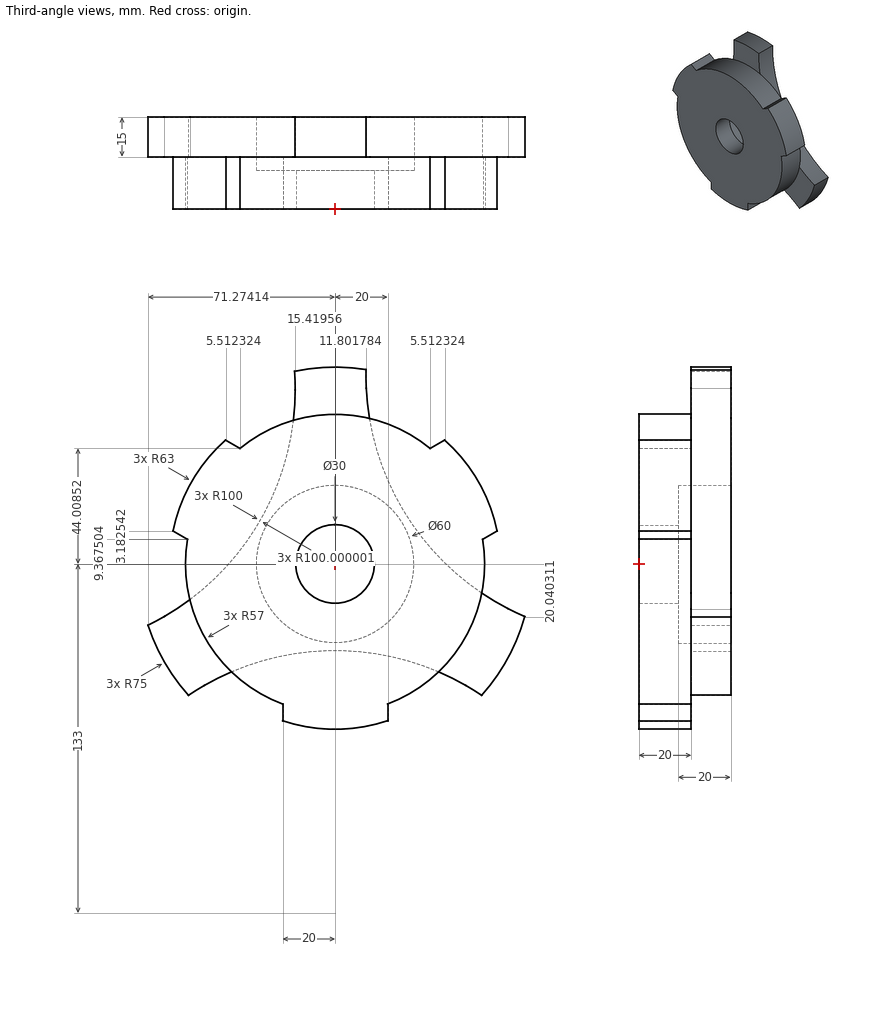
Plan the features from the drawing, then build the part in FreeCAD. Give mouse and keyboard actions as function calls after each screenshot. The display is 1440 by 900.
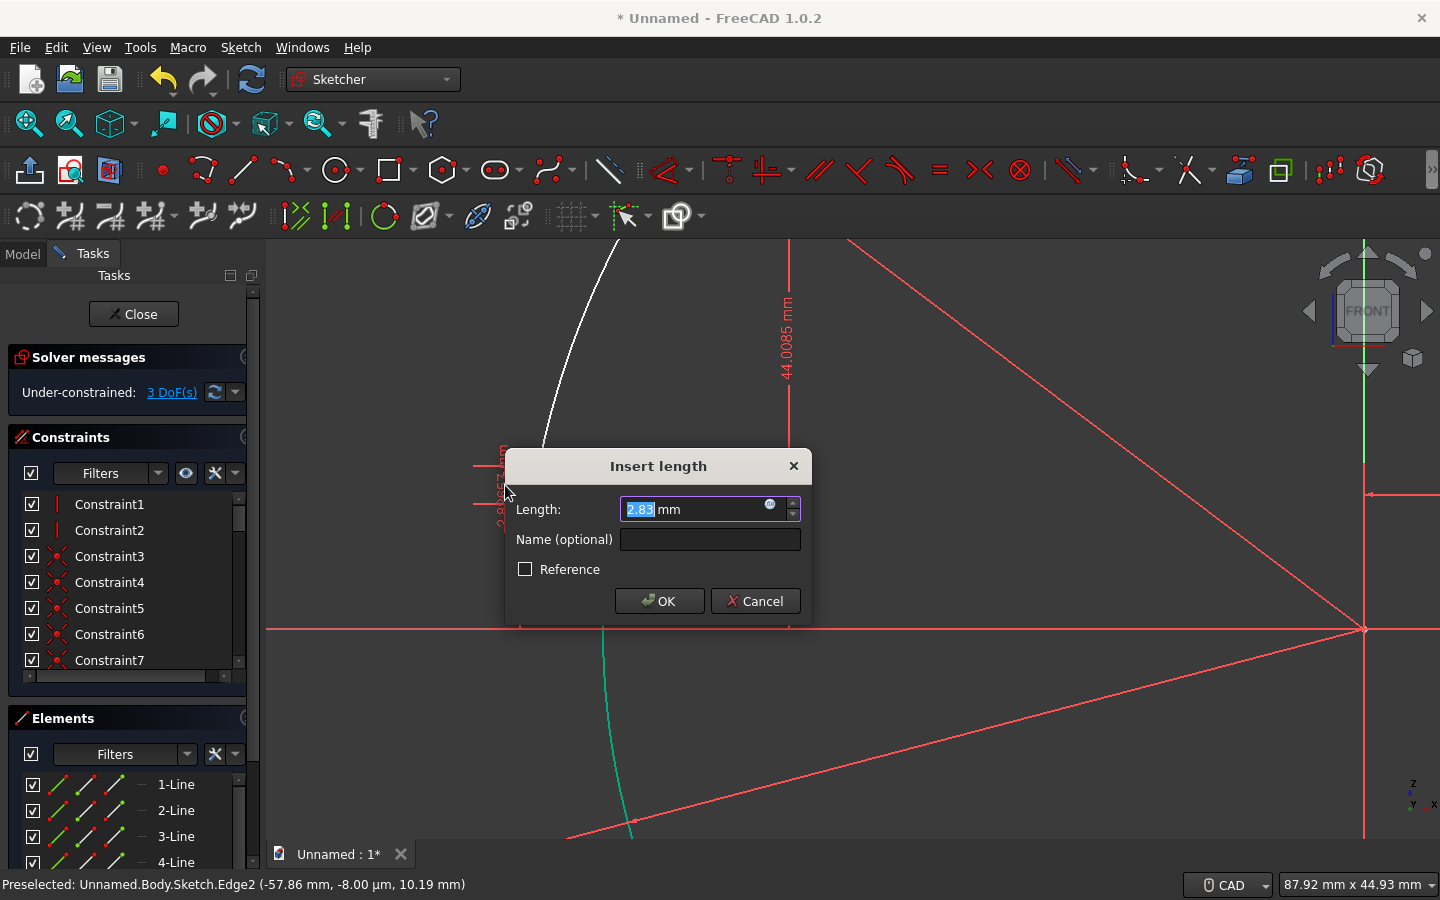
text(3.182542)
key(Return)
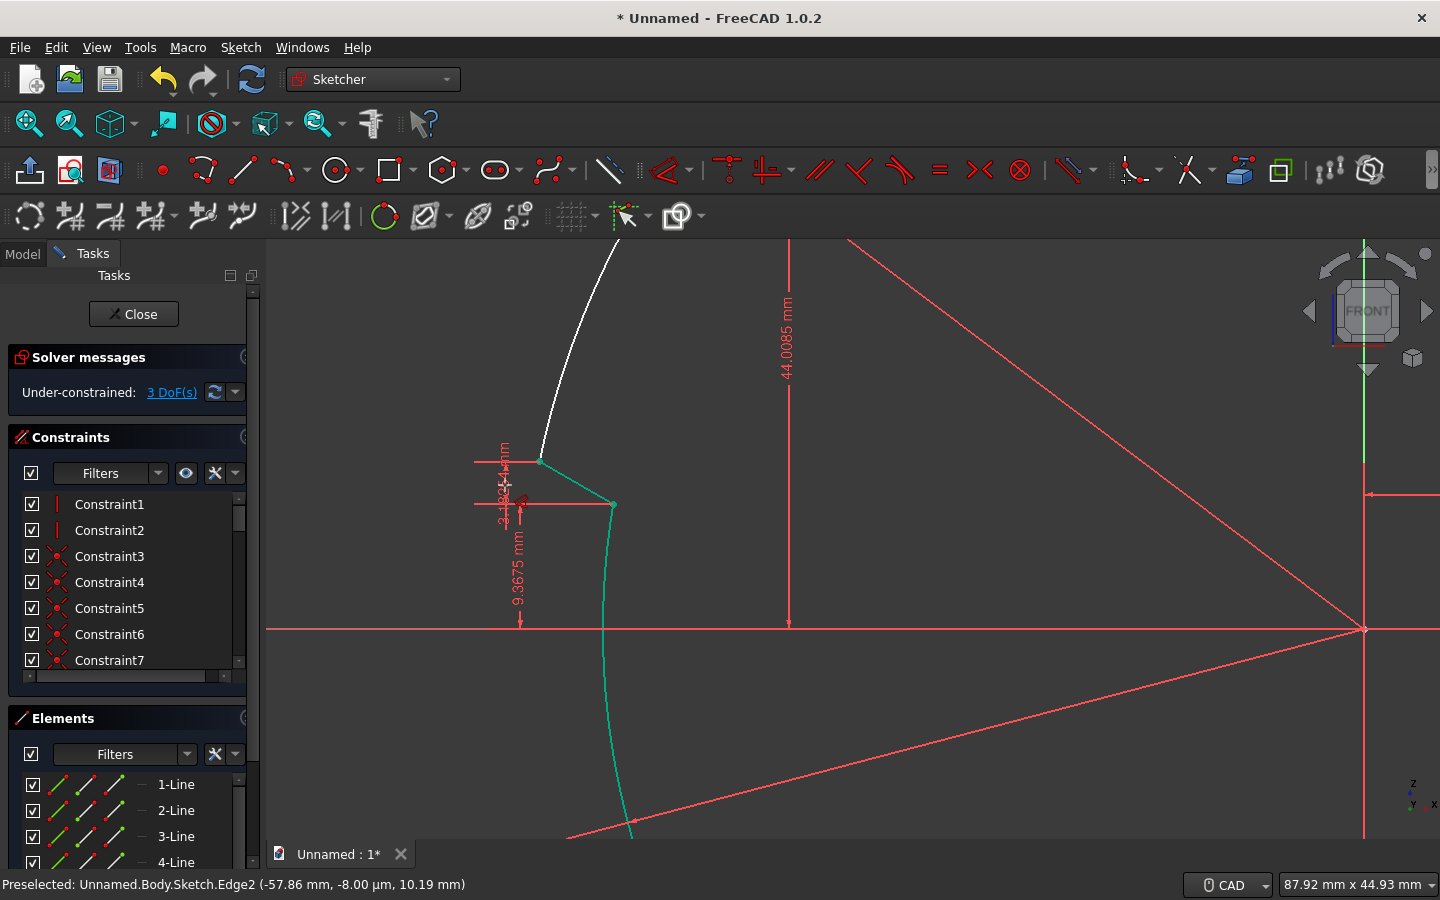
scroll(595, 496, down, 7)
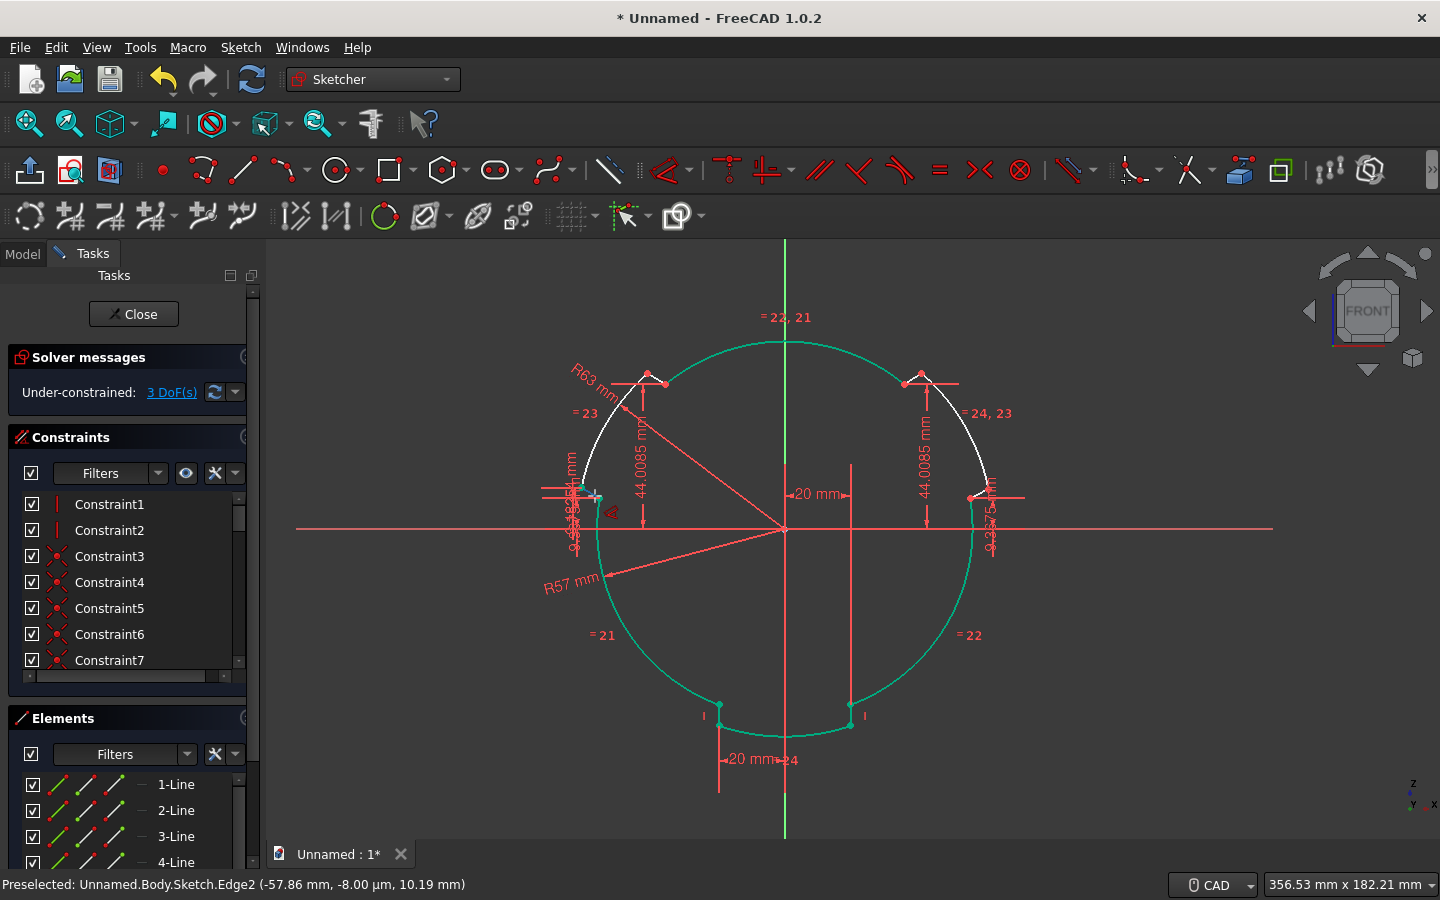
scroll(653, 377, up, 4)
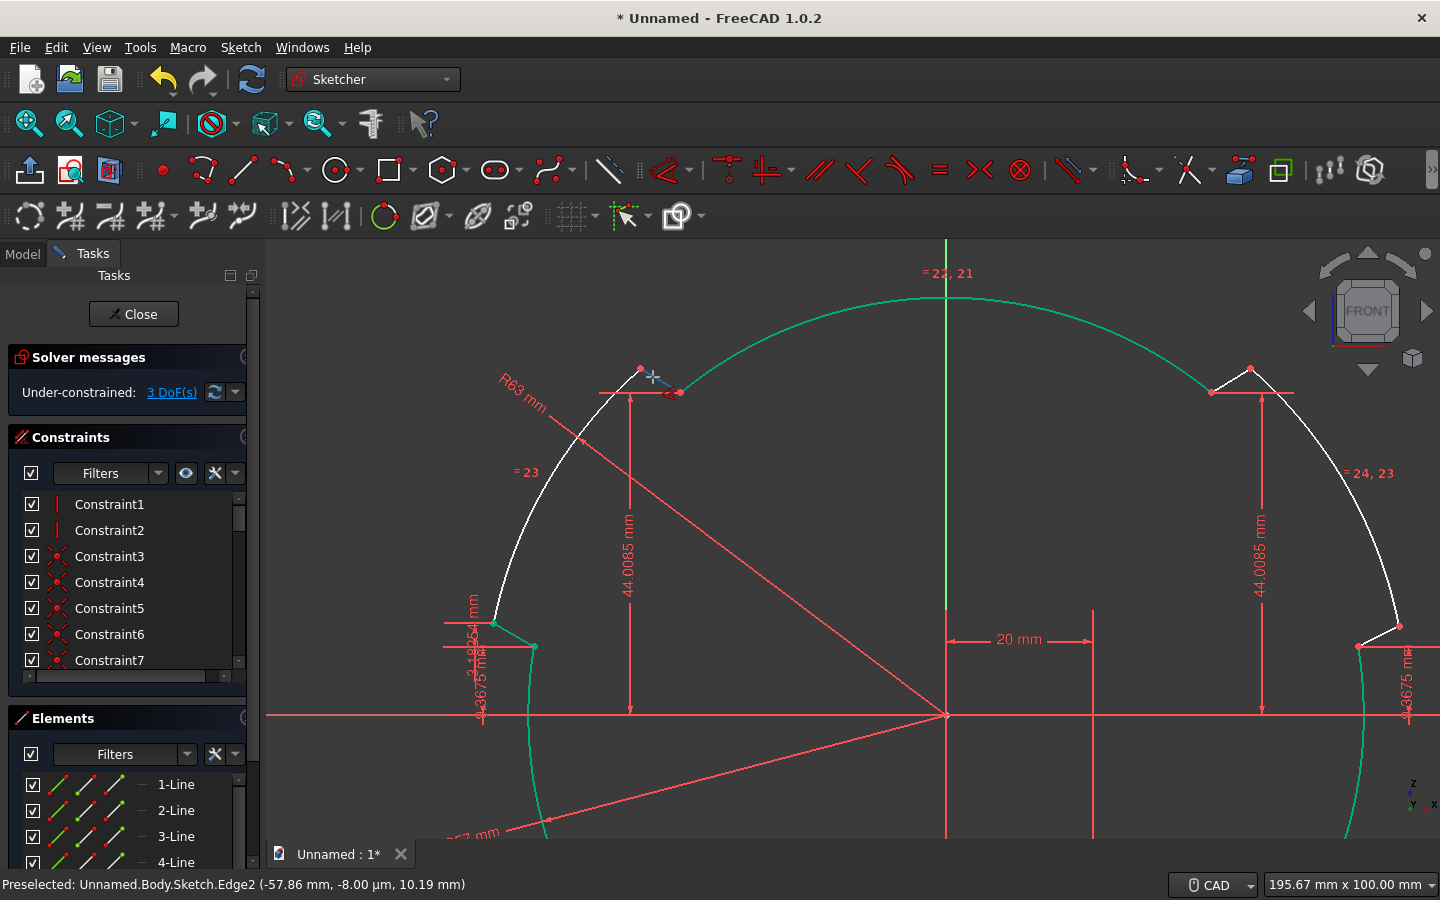
click(653, 376)
click(661, 335)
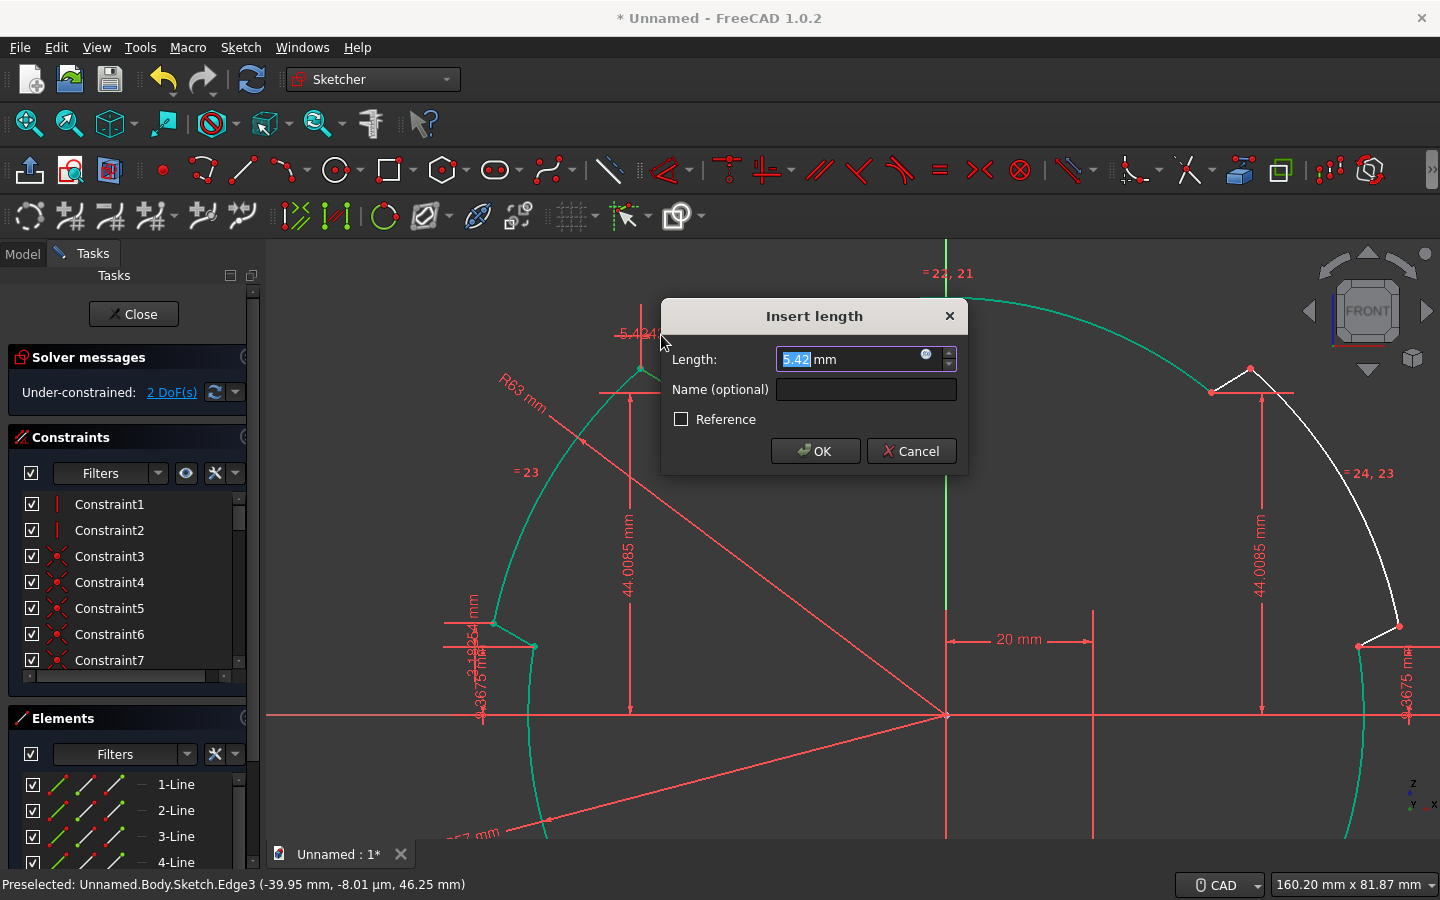
text(5.512324)
key(Return)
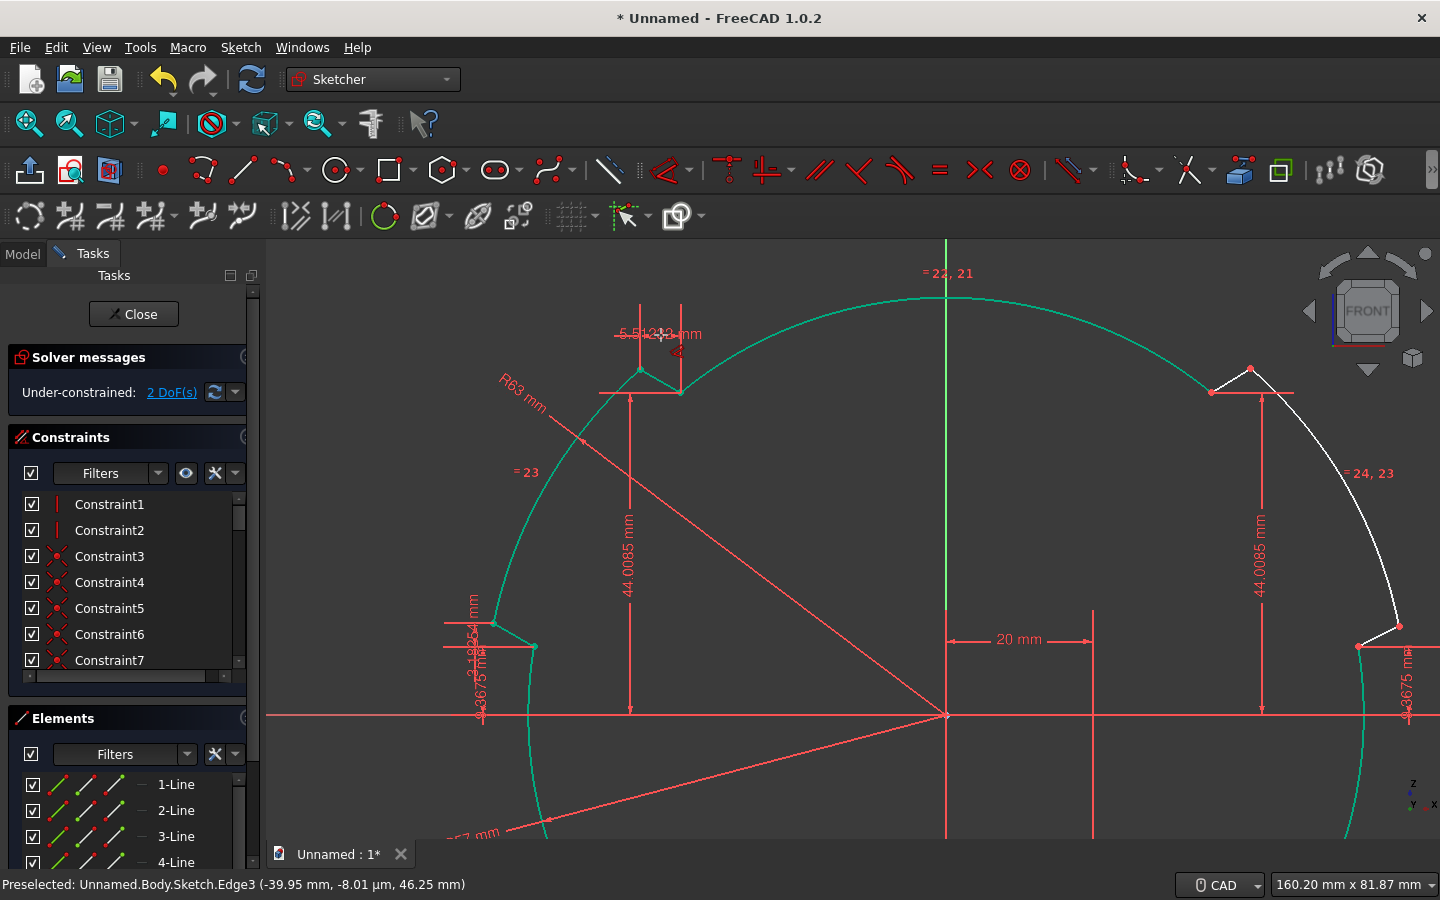
click(1223, 386)
click(1231, 335)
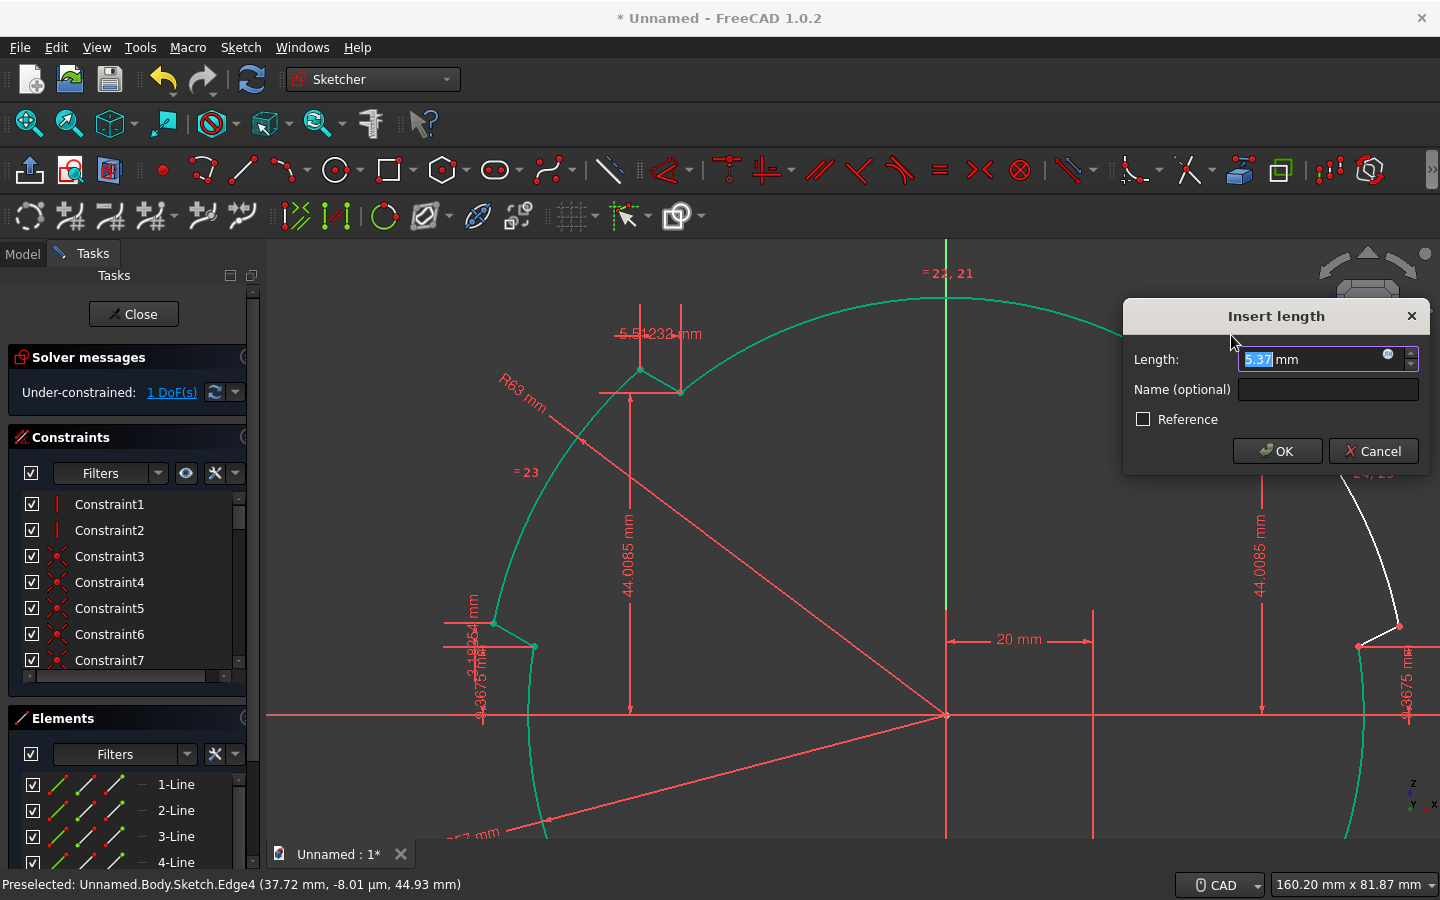
text(5.512324)
key(Return)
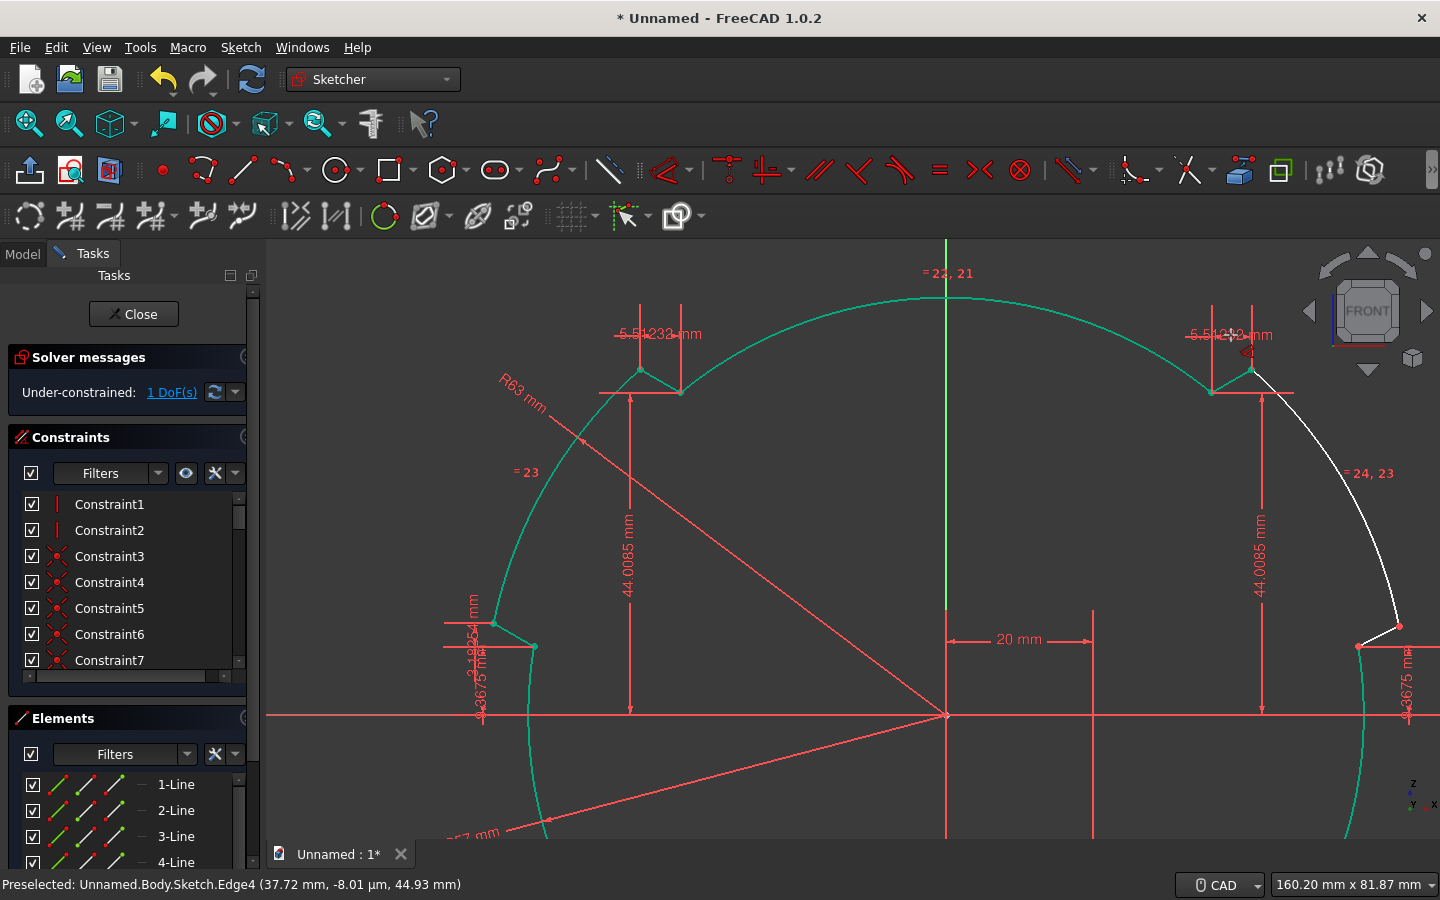
scroll(653, 377, down, 4)